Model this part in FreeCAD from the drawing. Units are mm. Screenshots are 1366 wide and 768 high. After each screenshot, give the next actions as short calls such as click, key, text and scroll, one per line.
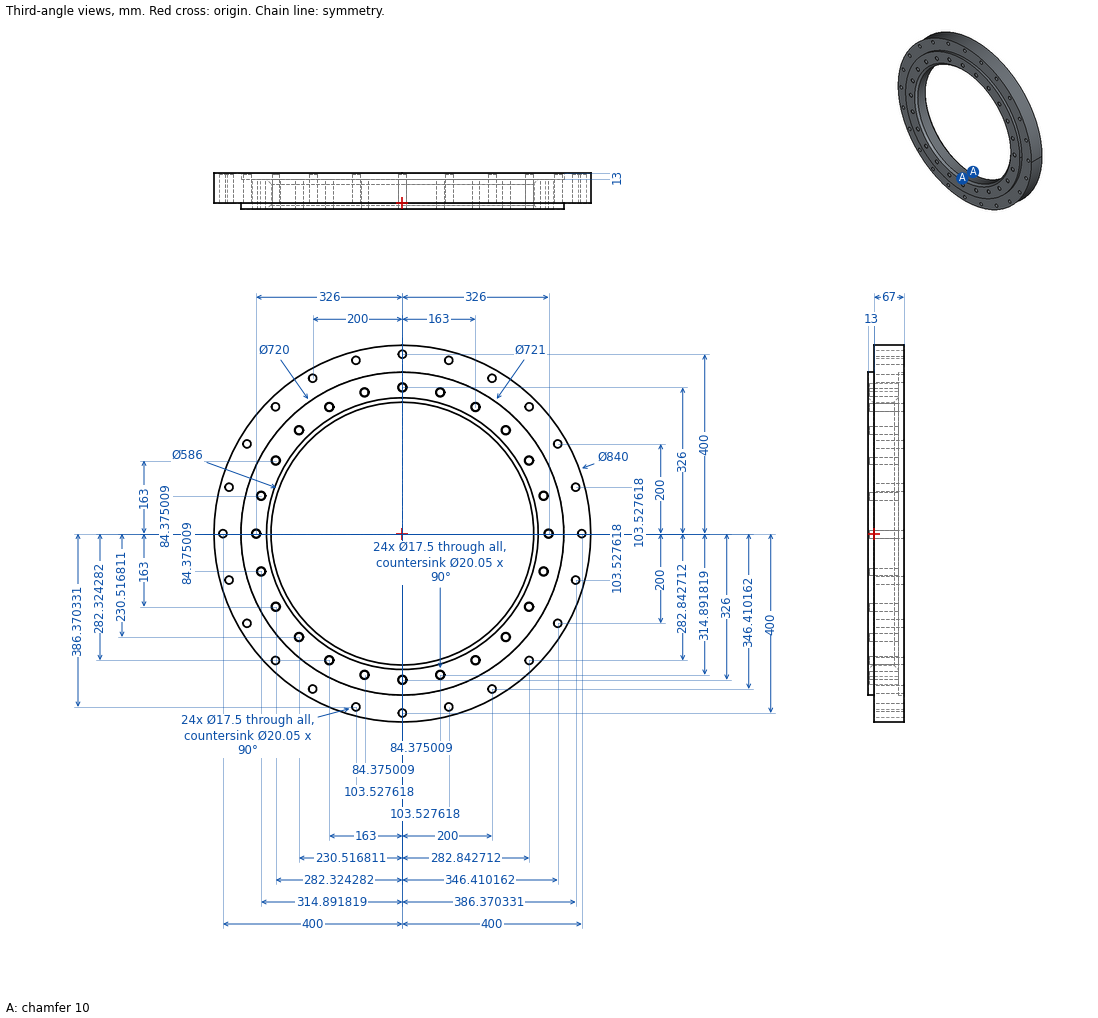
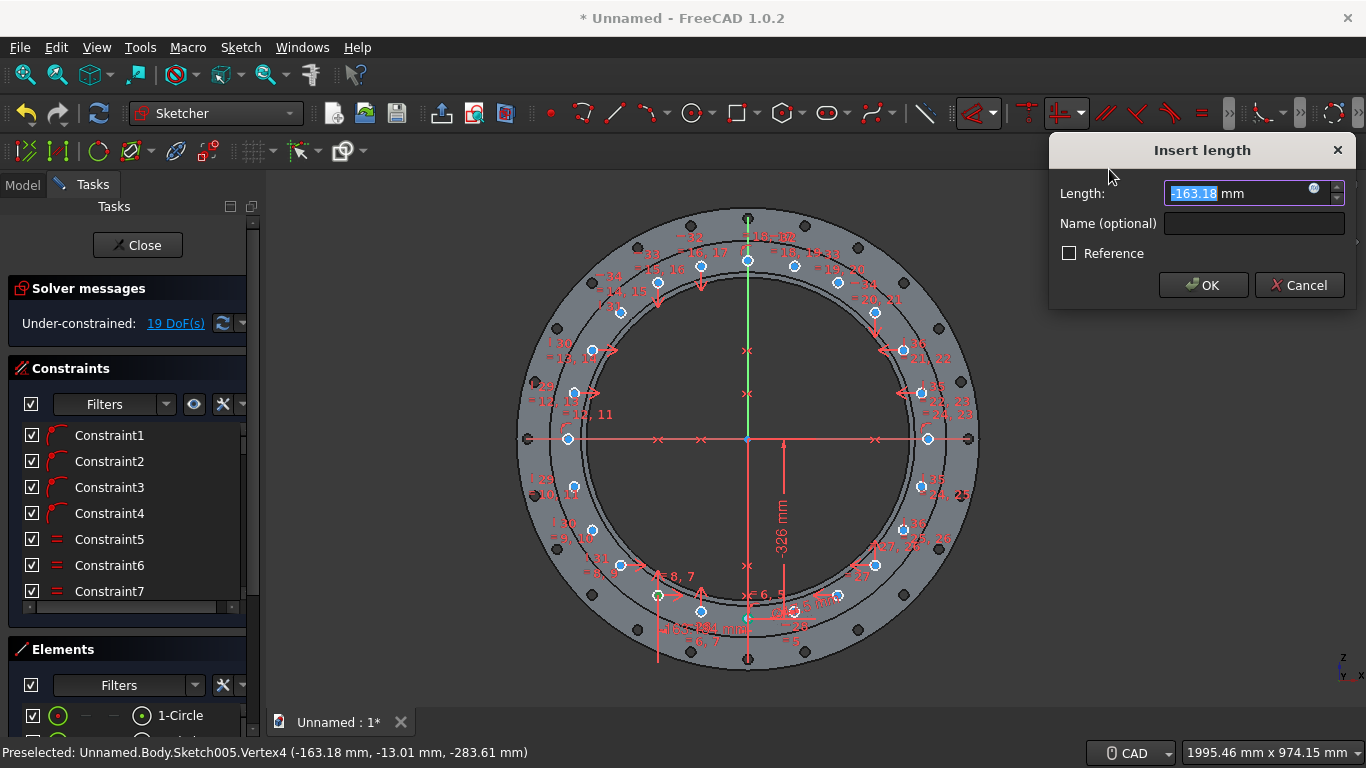
text(-163)
key(Return)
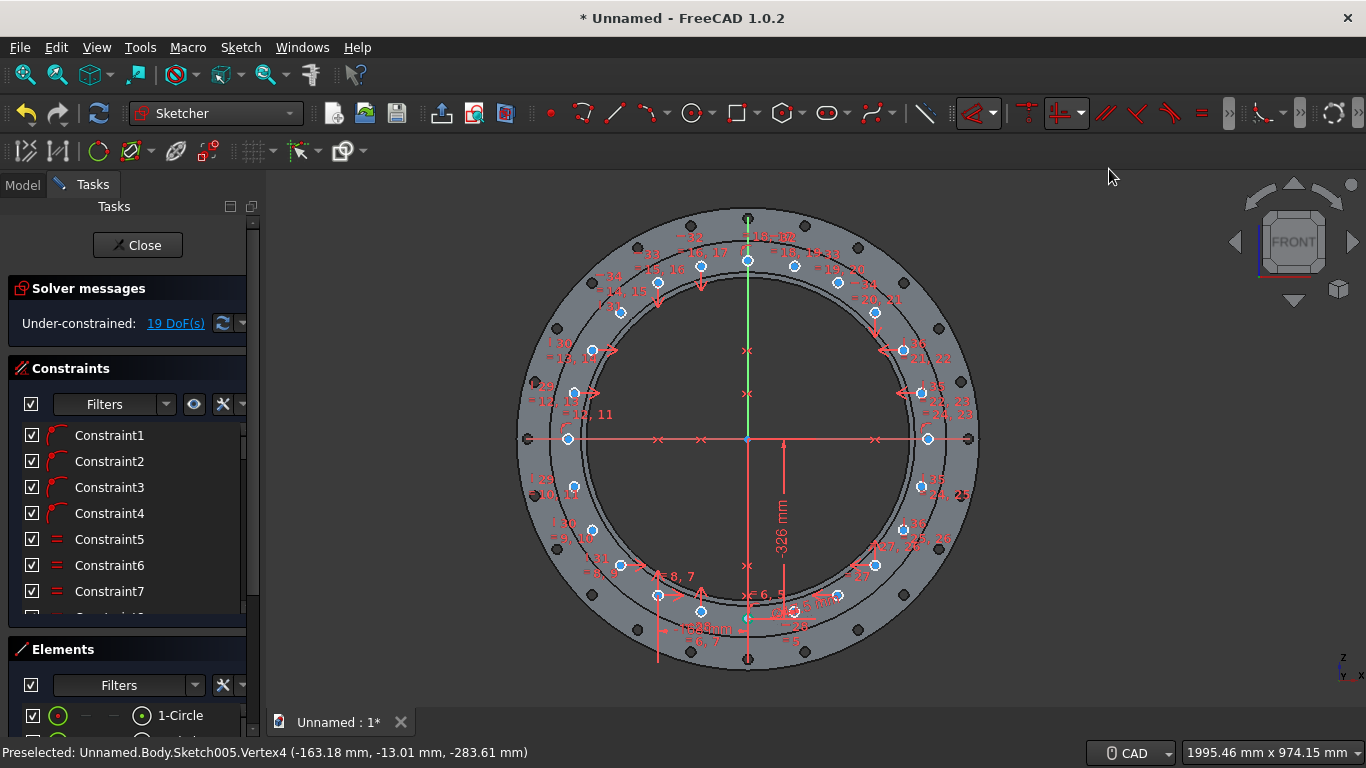
click(592, 530)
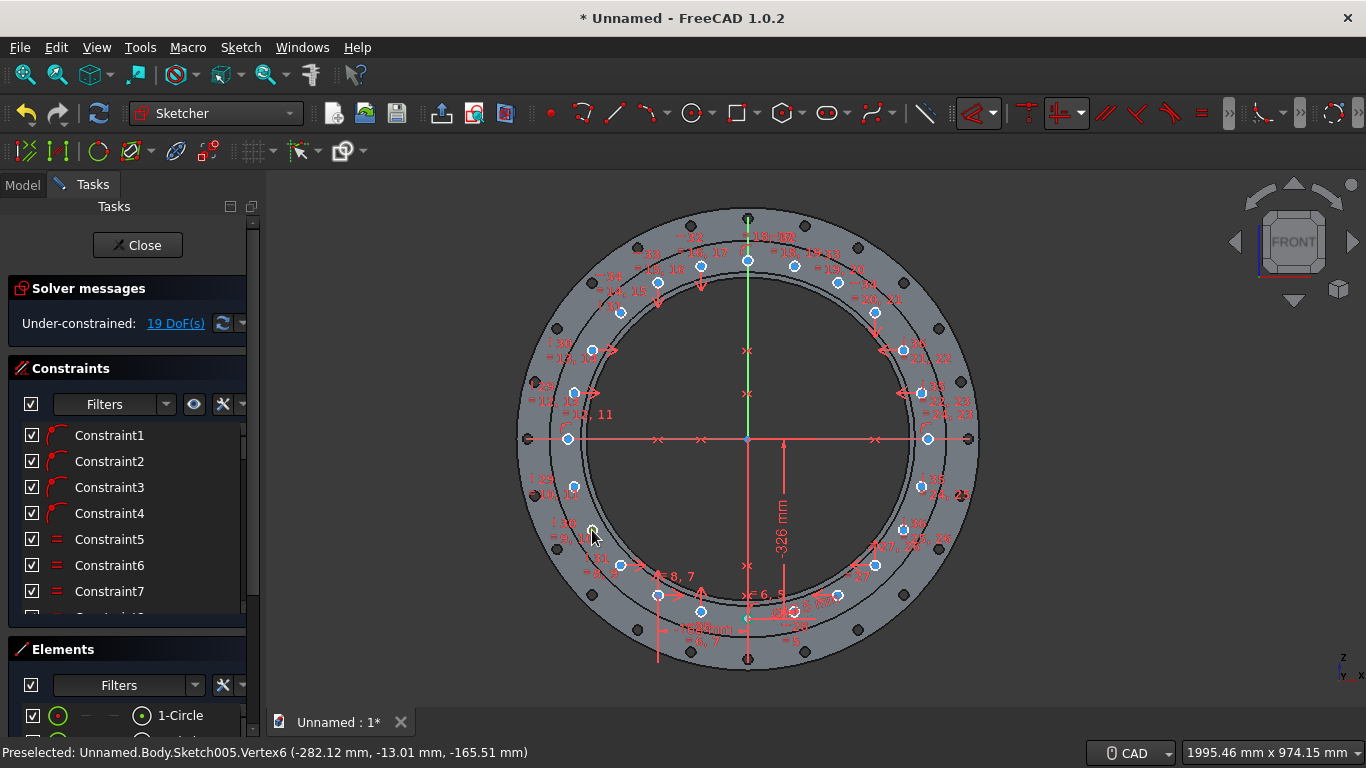
click(996, 114)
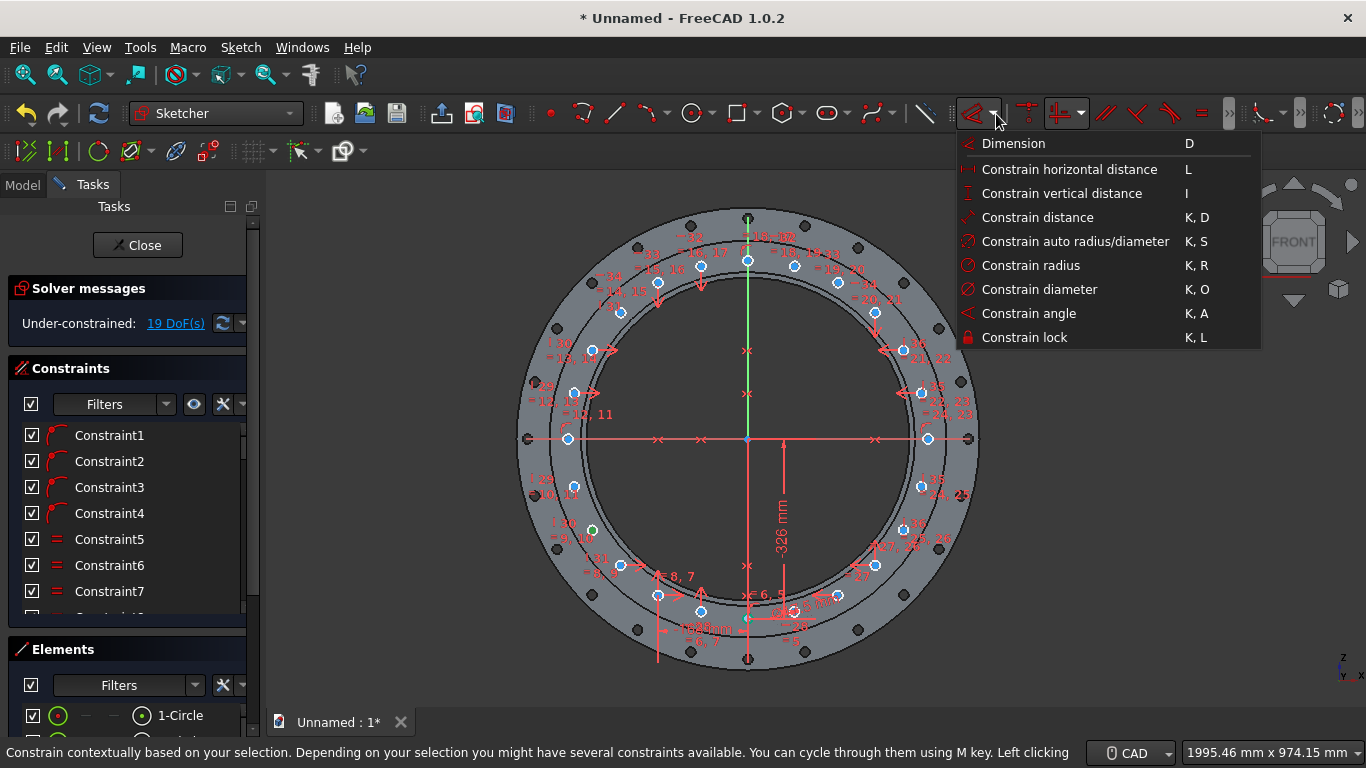
click(1109, 193)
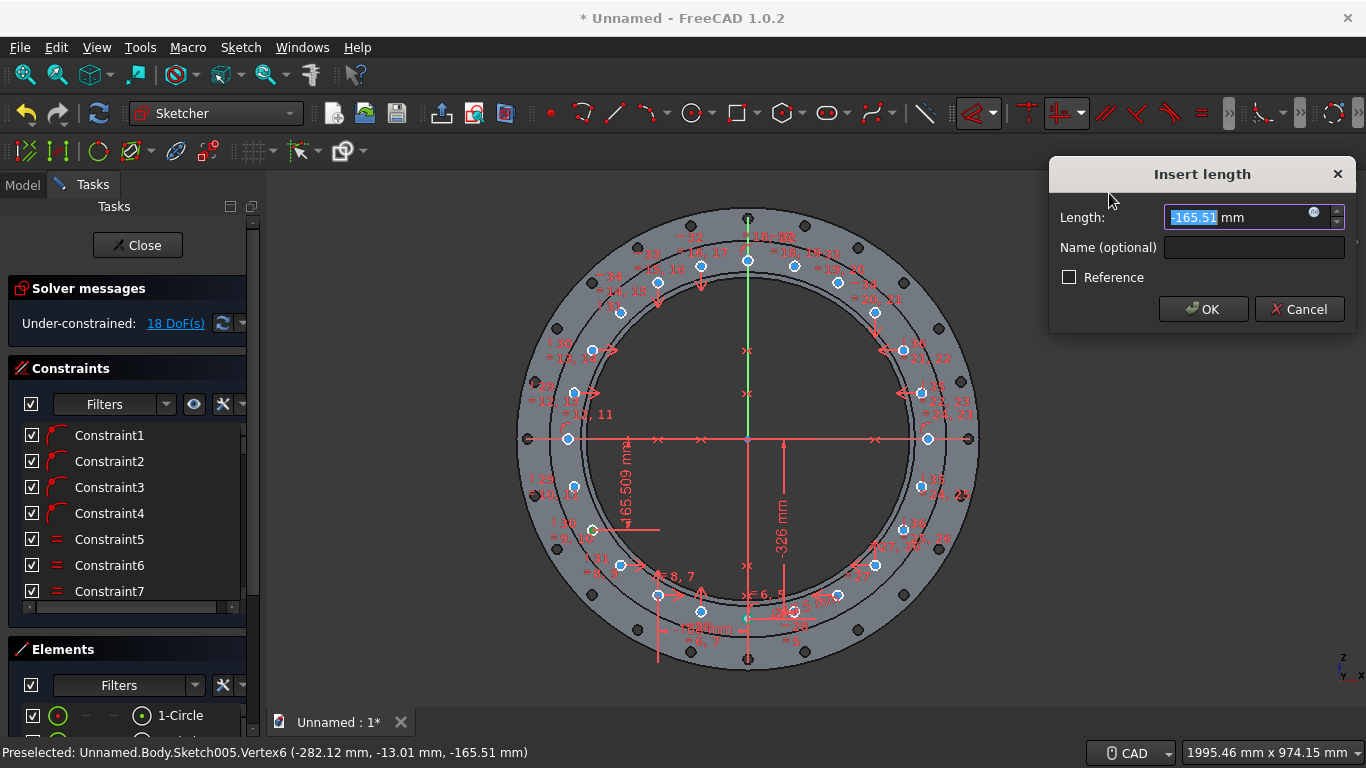
text(-163)
key(Return)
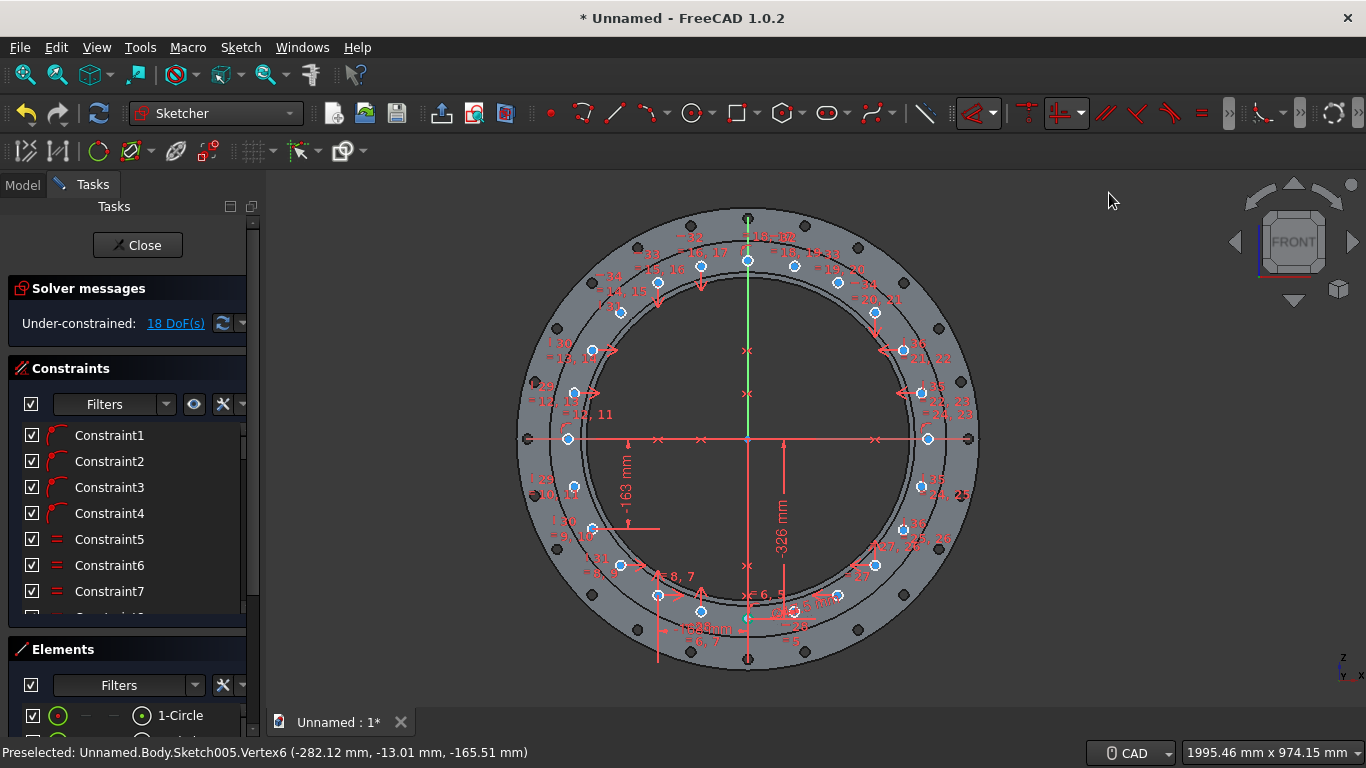
click(568, 439)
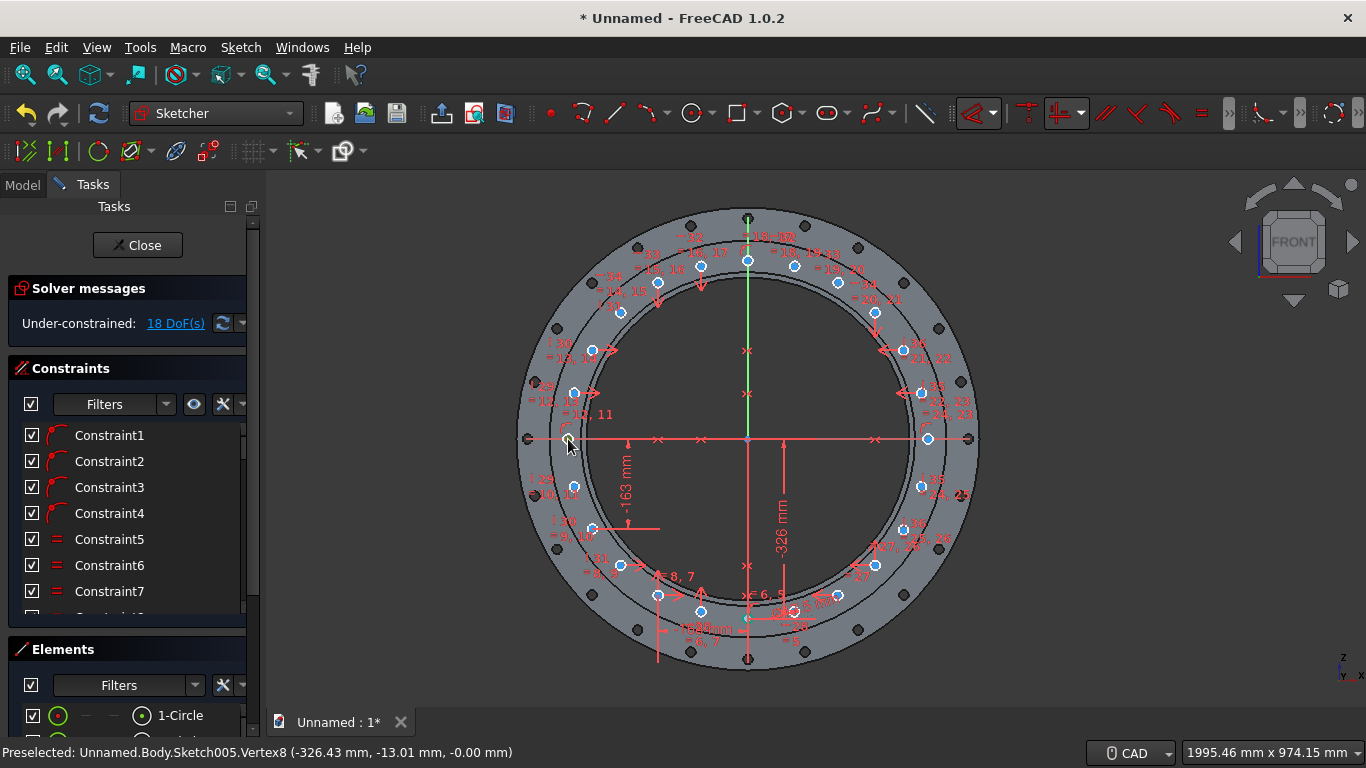
click(996, 114)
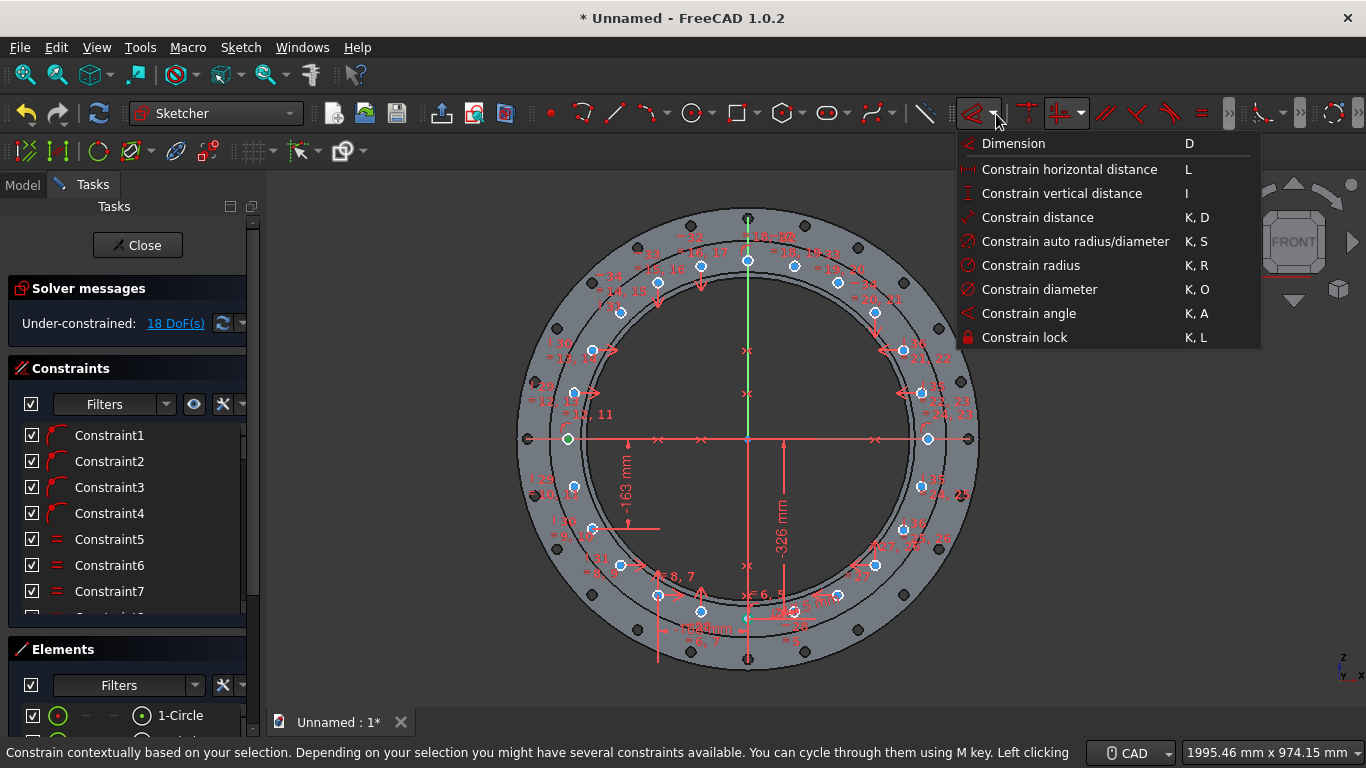
click(1109, 169)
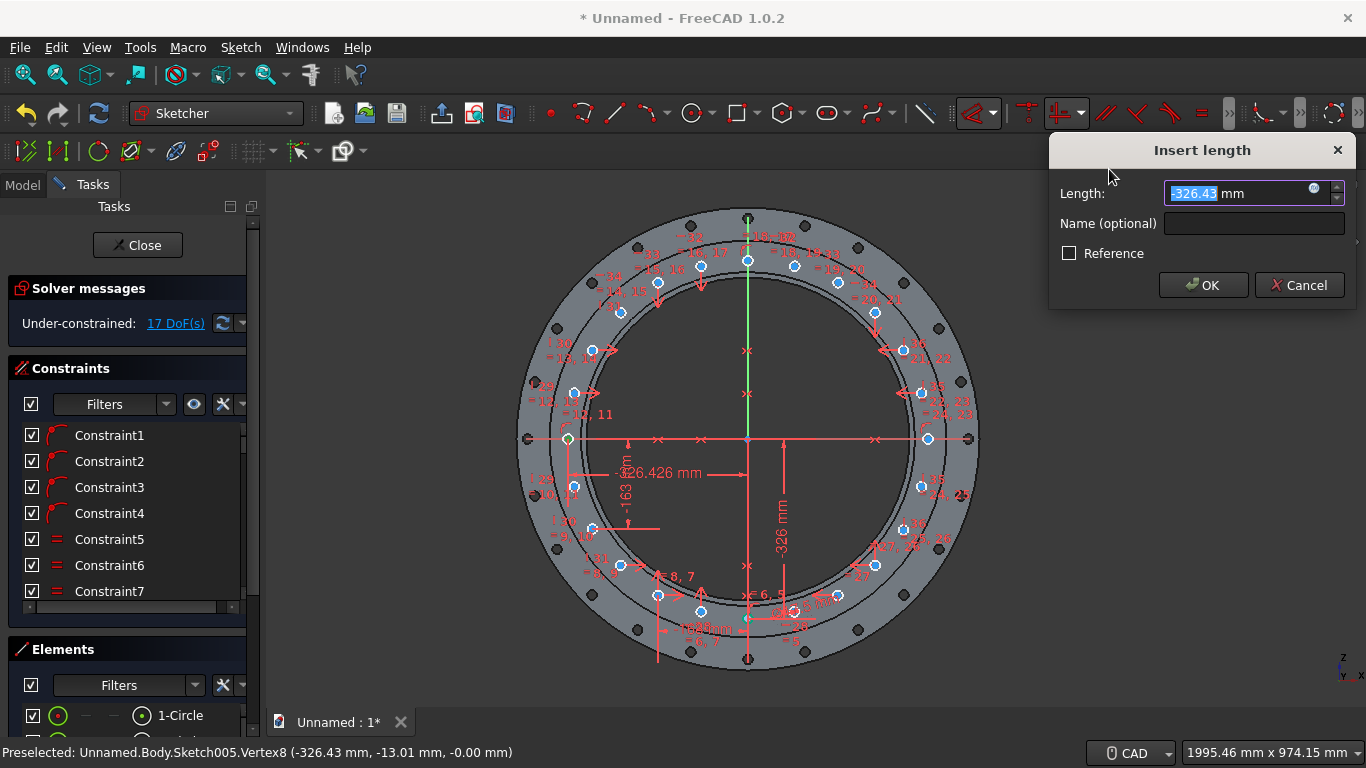
text(-326)
key(Return)